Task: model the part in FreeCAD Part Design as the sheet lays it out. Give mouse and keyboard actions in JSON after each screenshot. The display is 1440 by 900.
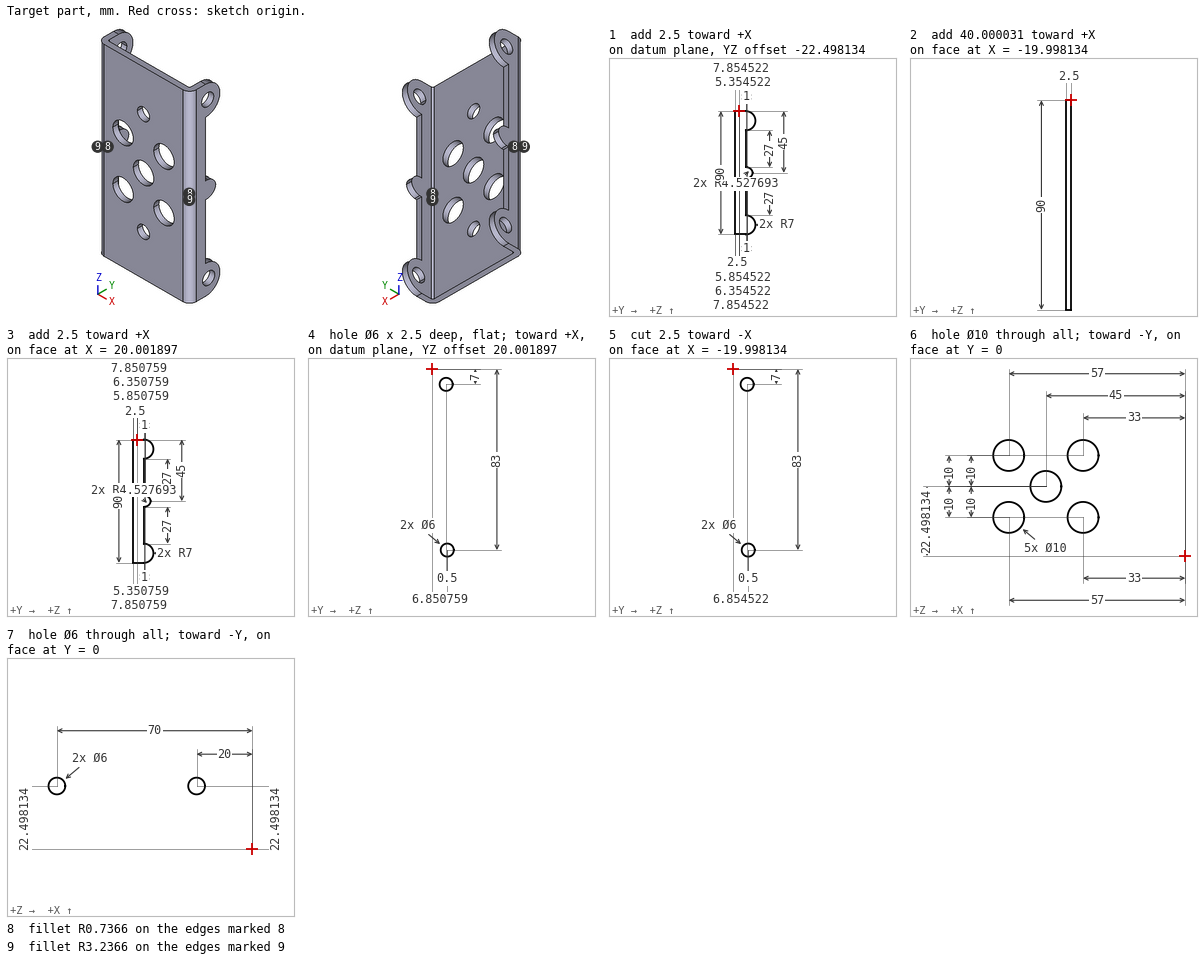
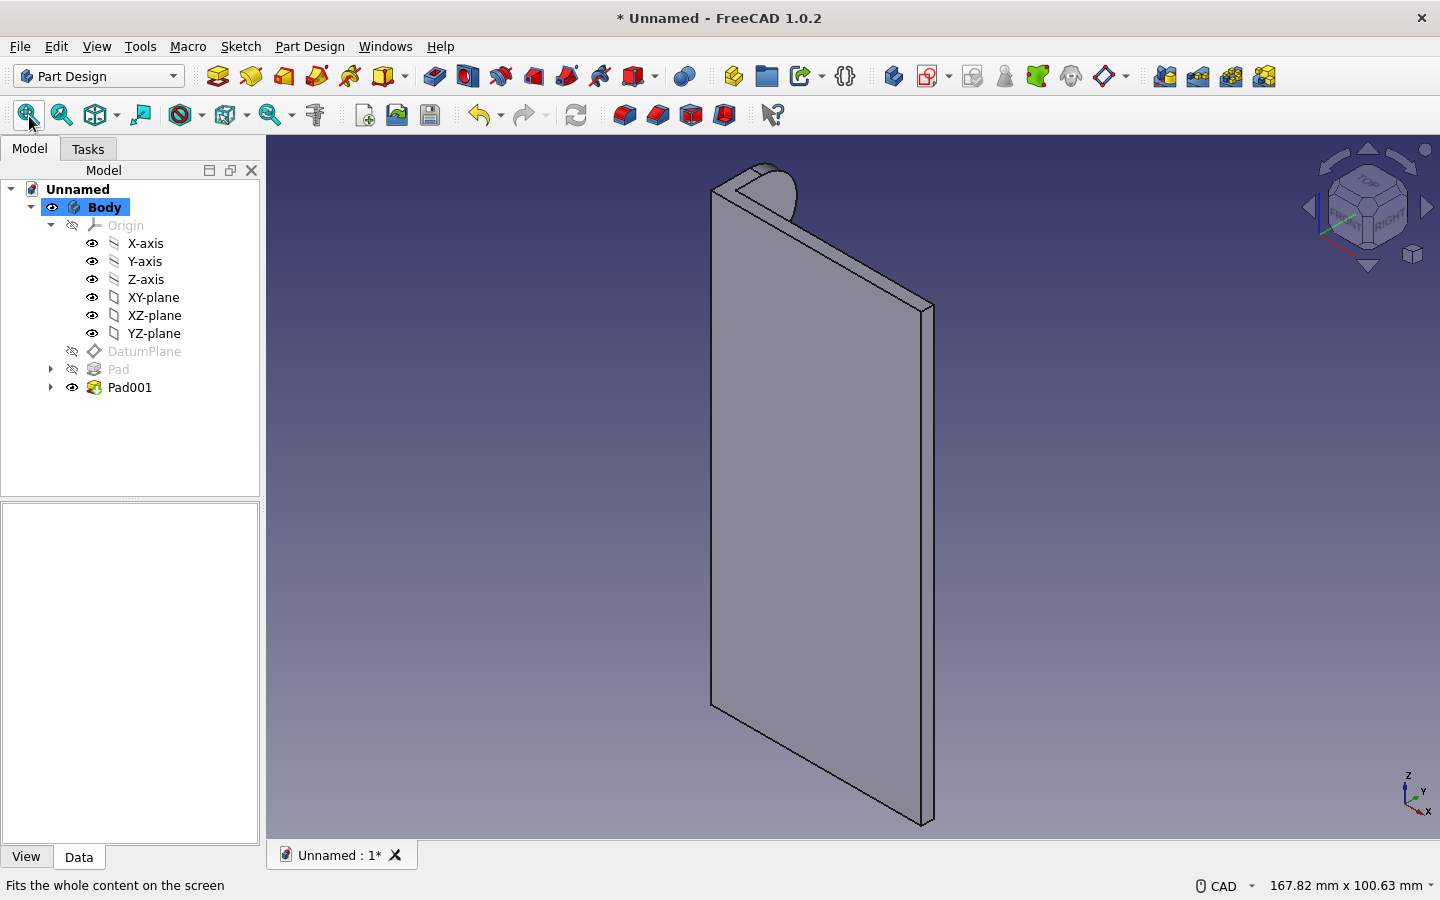
{"action": "key", "text": "3"}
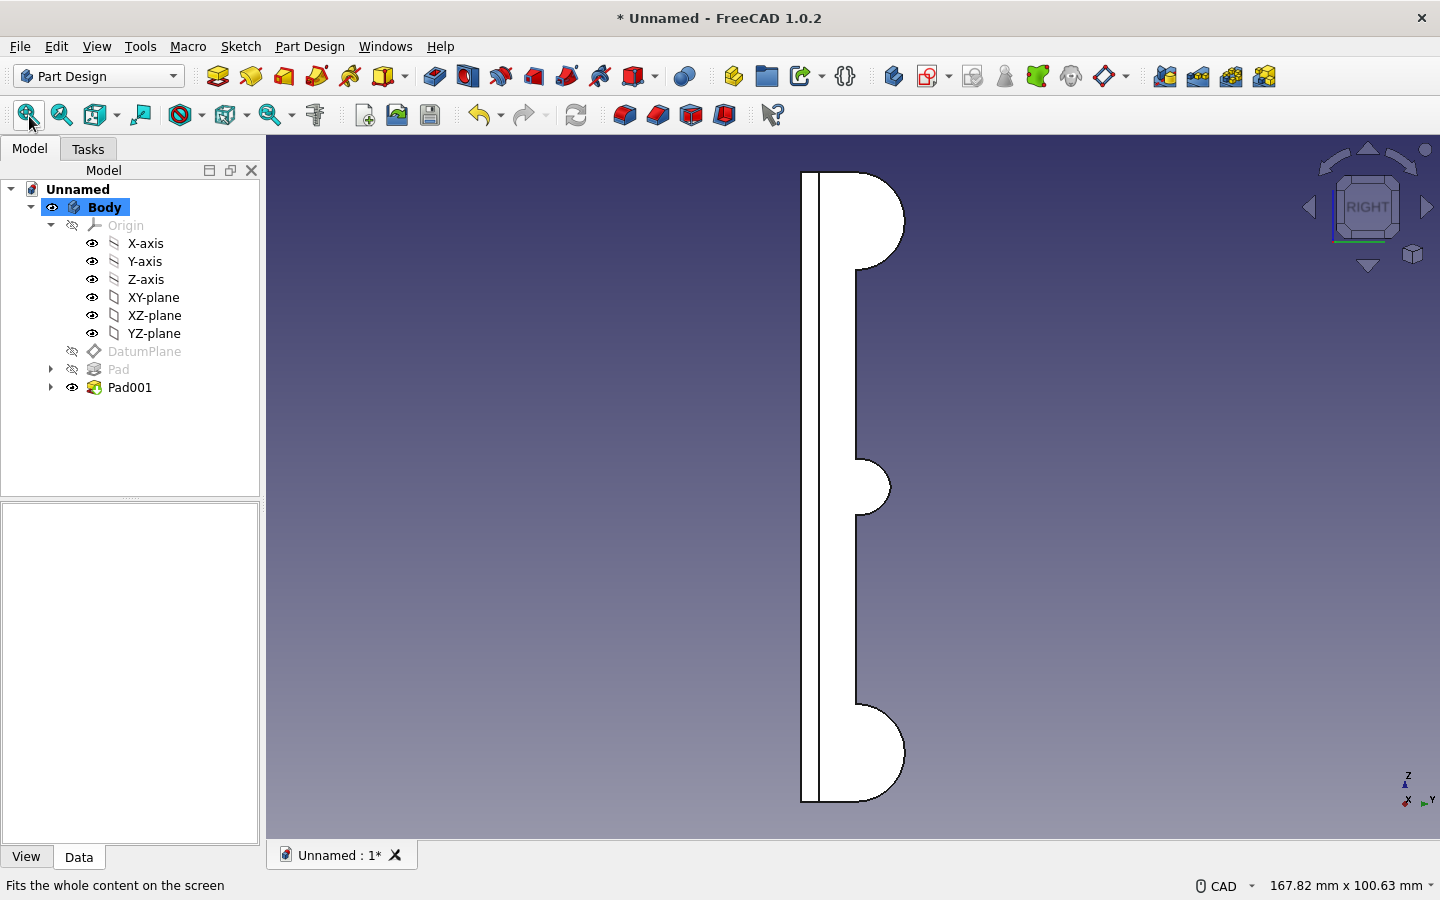
{"action": "left_click", "coordinate": [810, 216]}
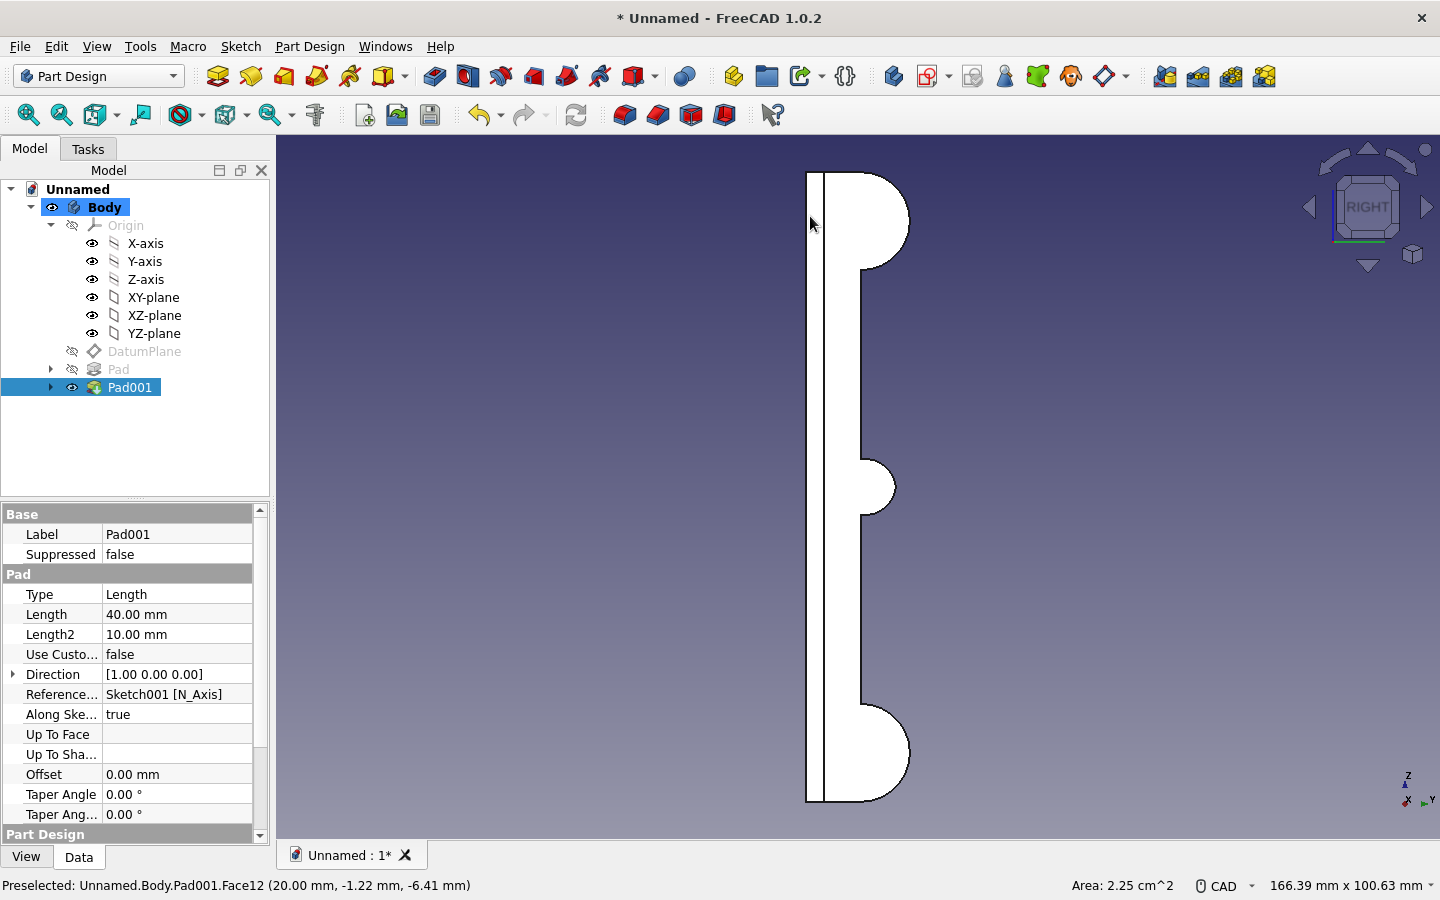
{"action": "left_click", "coordinate": [926, 76]}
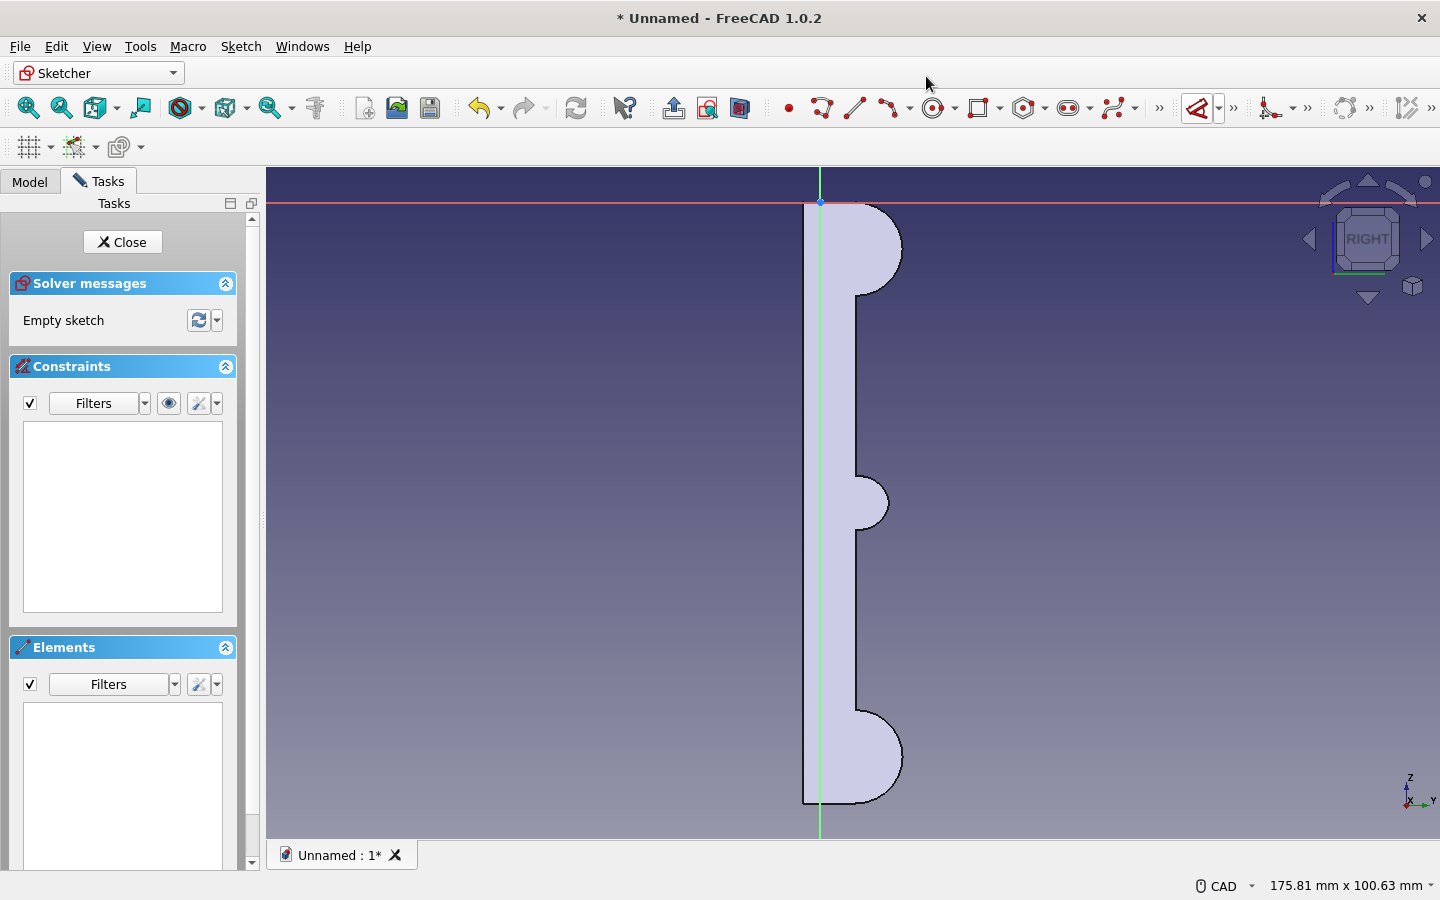
{"action": "scroll", "coordinate": [645, 503], "scroll_direction": "down", "scroll_amount": 2}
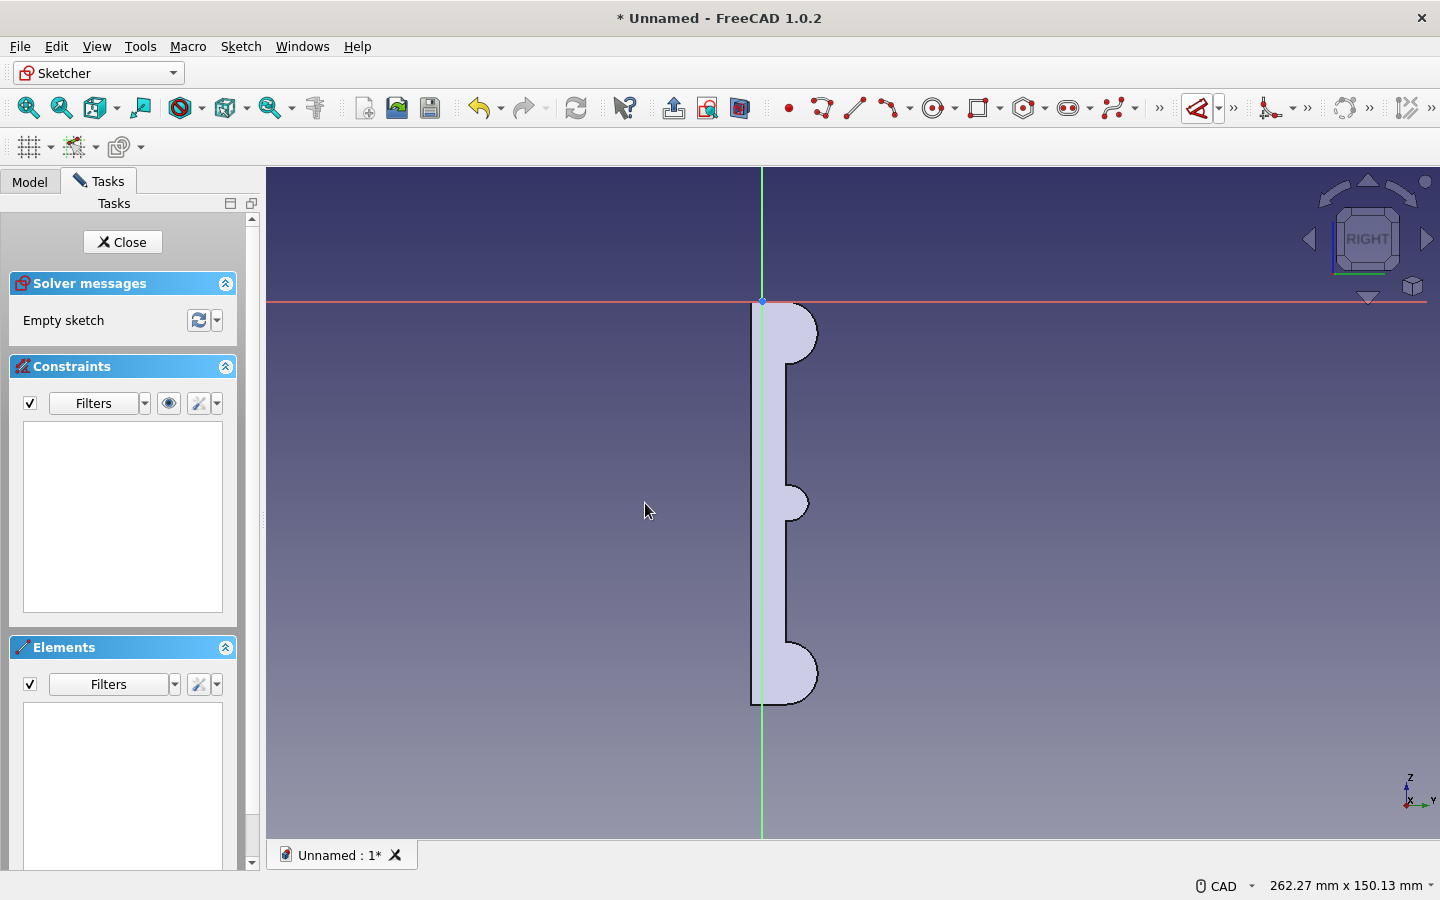
{"action": "left_click", "coordinate": [822, 108]}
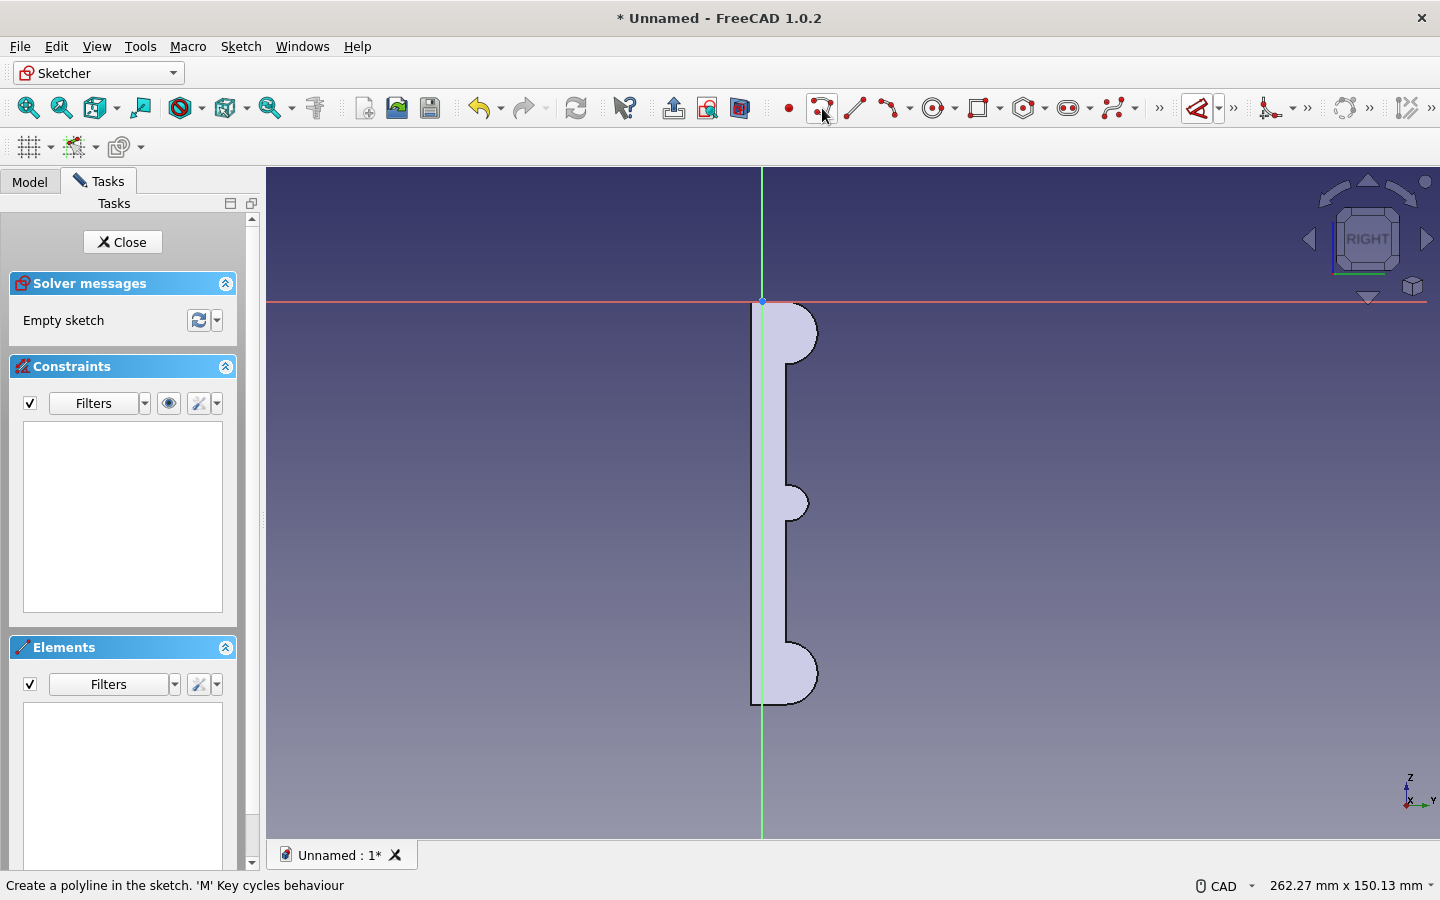
{"action": "left_click", "coordinate": [786, 302]}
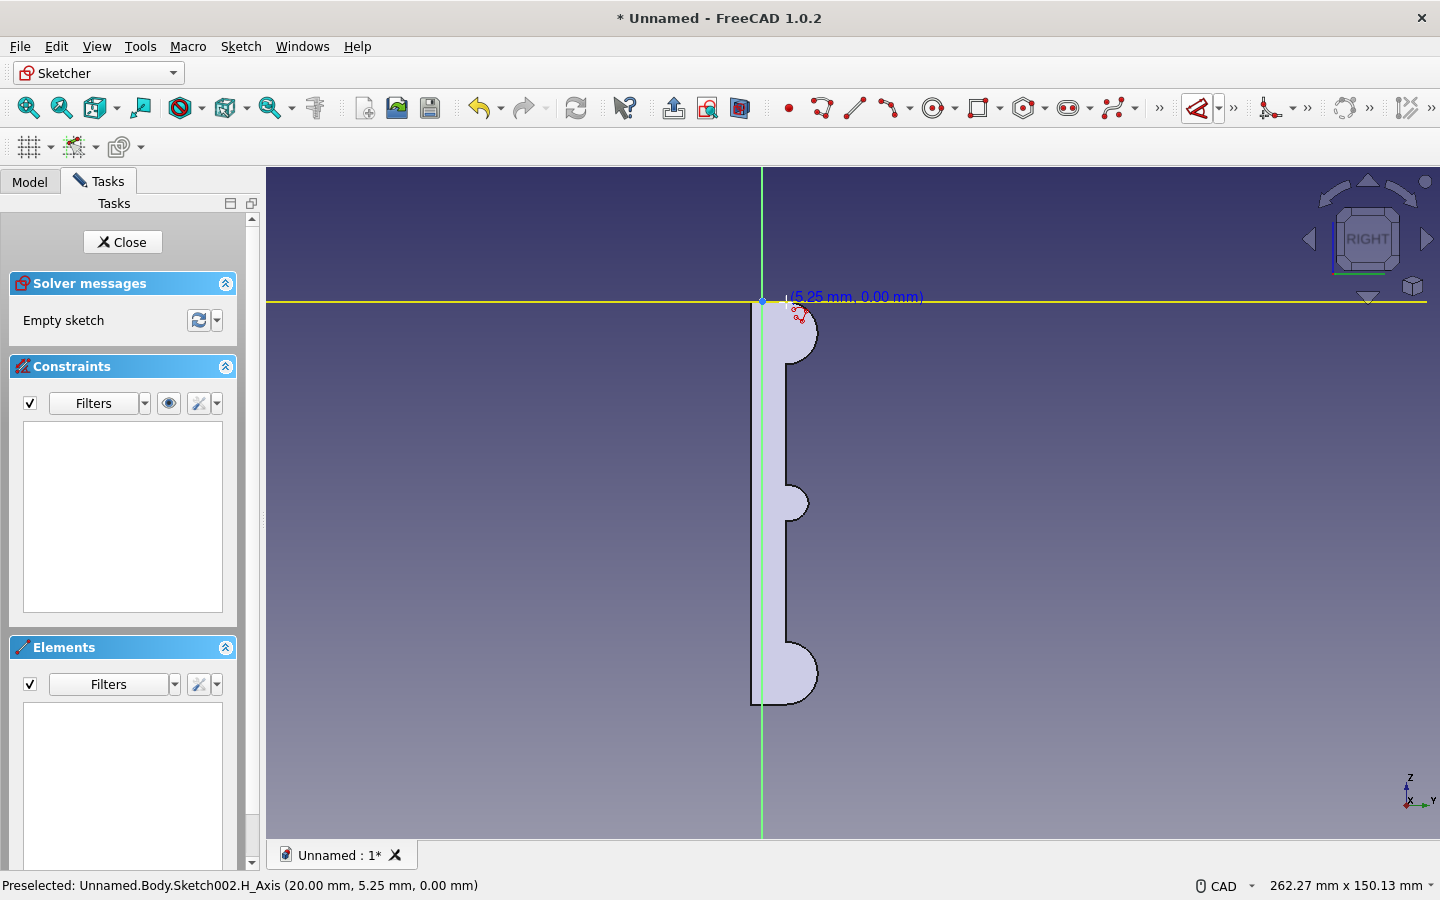
{"action": "scroll", "coordinate": [751, 302], "scroll_direction": "up", "scroll_amount": 2}